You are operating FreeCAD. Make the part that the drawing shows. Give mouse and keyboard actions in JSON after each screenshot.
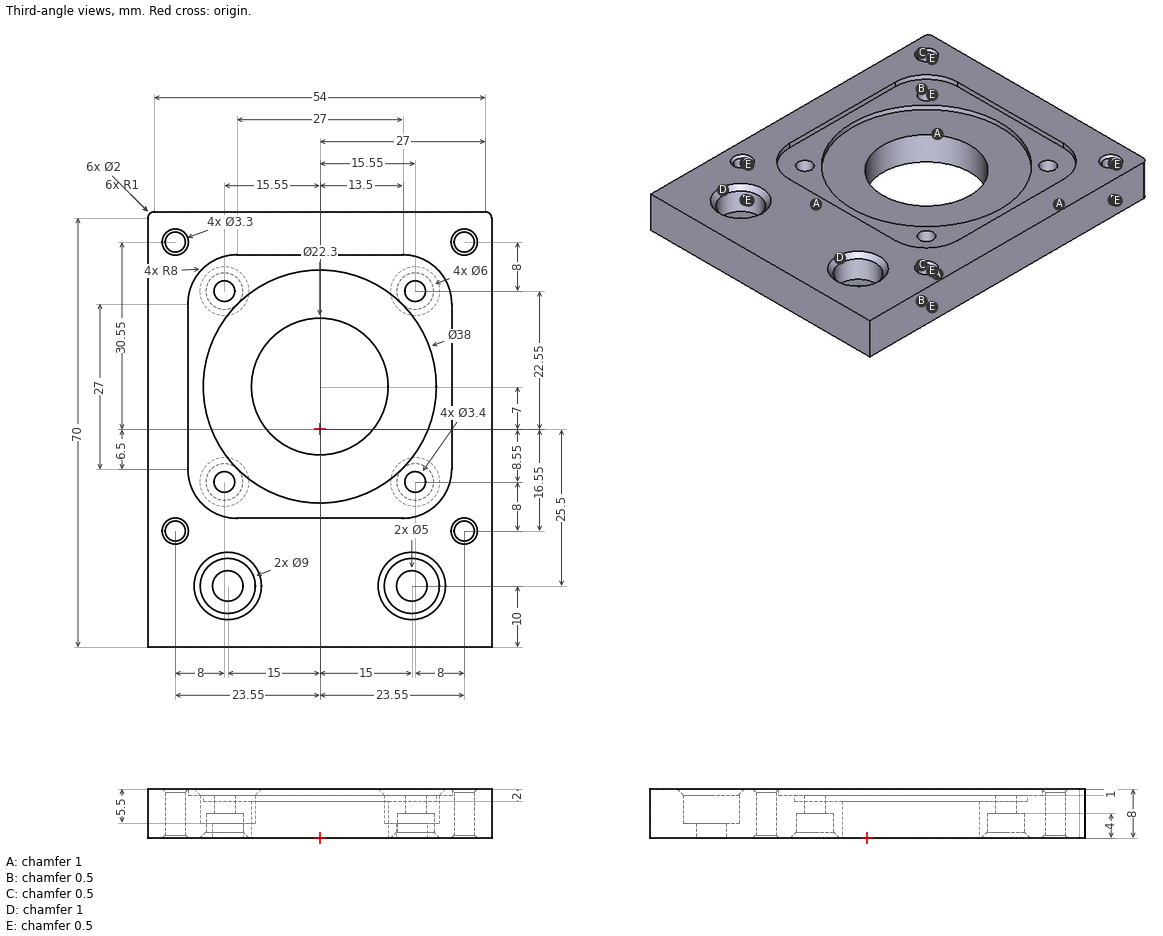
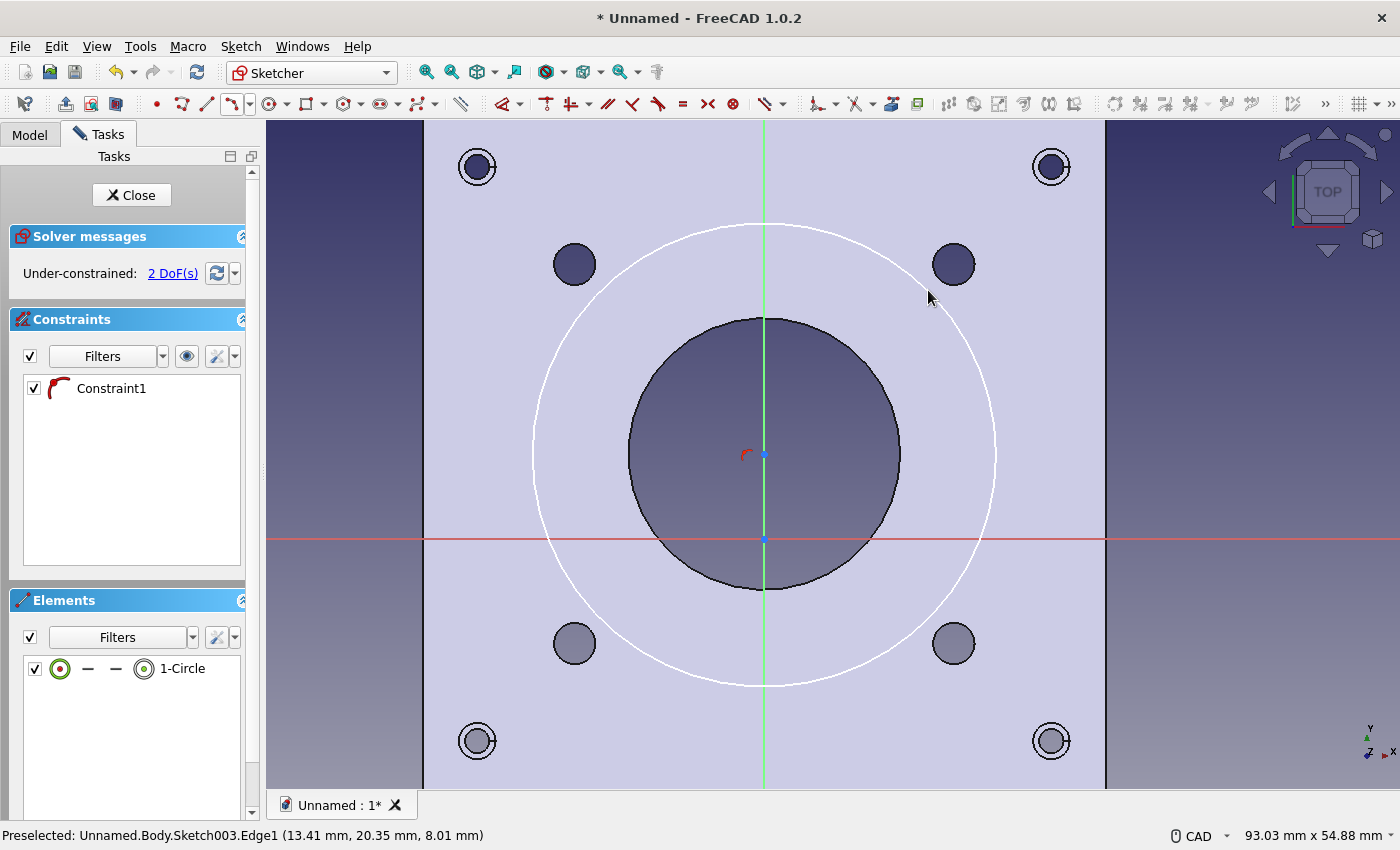
{"action": "key", "text": "d"}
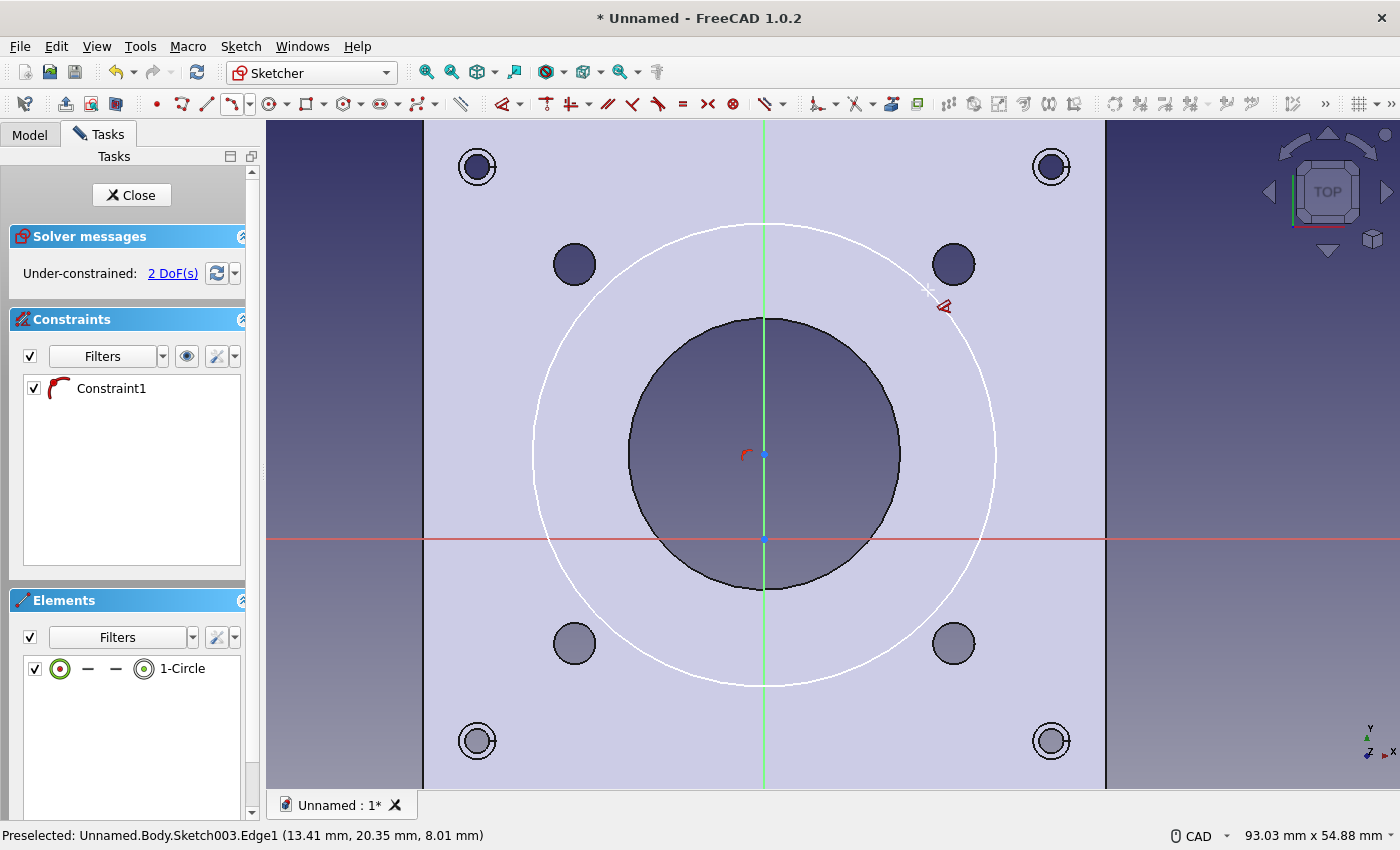
{"action": "left_click", "coordinate": [928, 291]}
{"action": "left_click", "coordinate": [951, 268]}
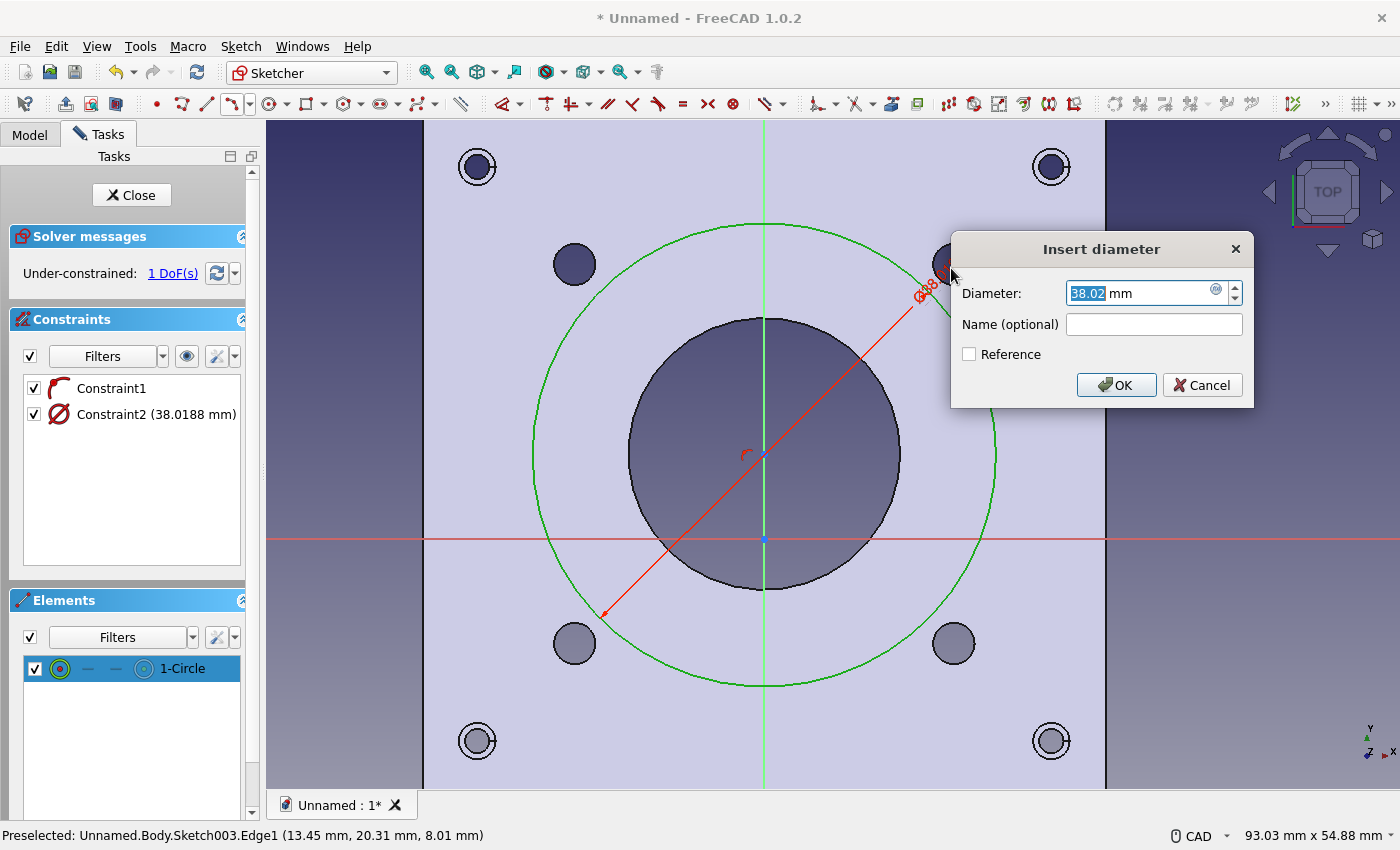
{"action": "type", "text": "38"}
{"action": "key", "text": "Return"}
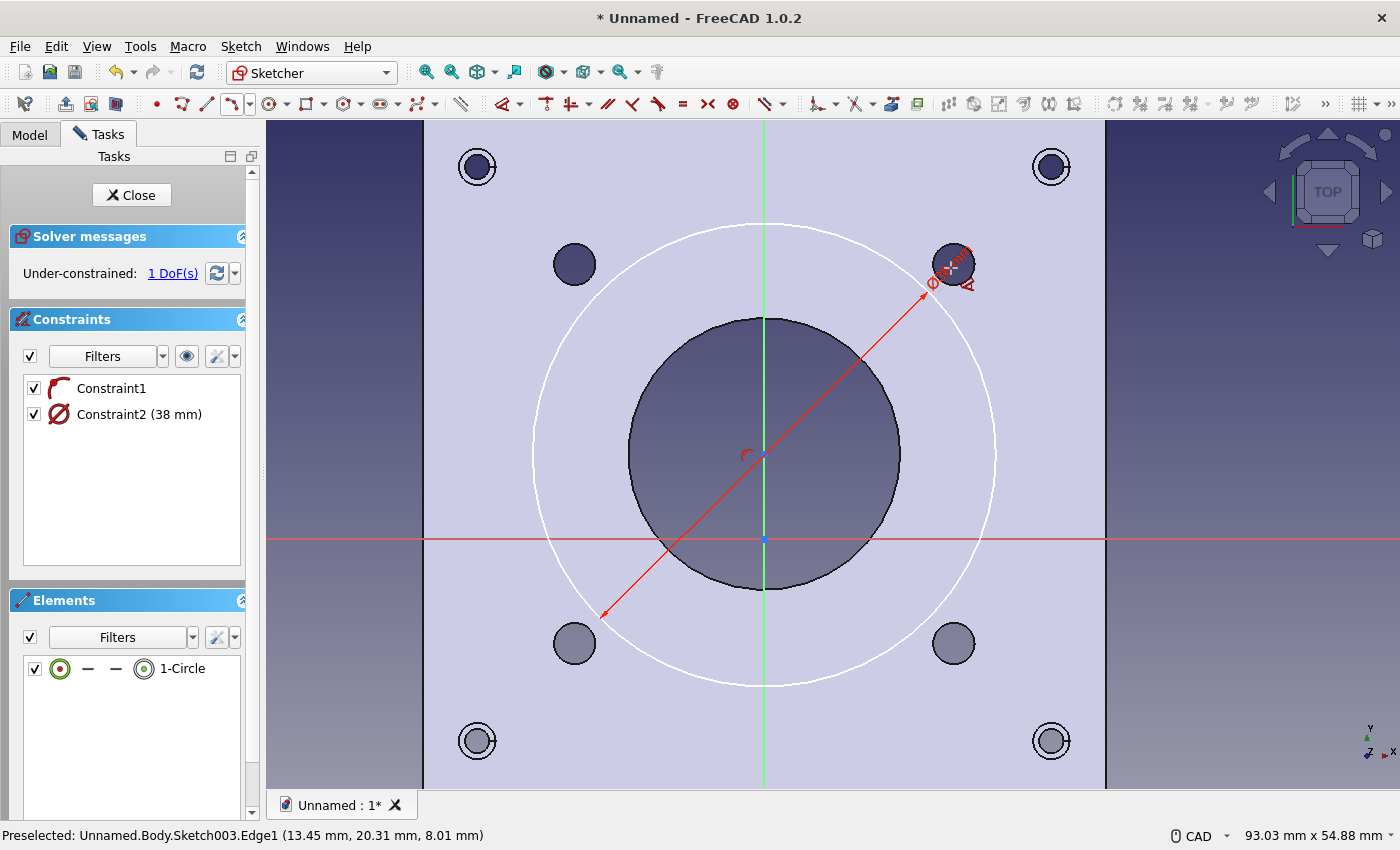
{"action": "left_click", "coordinate": [764, 455]}
{"action": "left_click", "coordinate": [798, 497]}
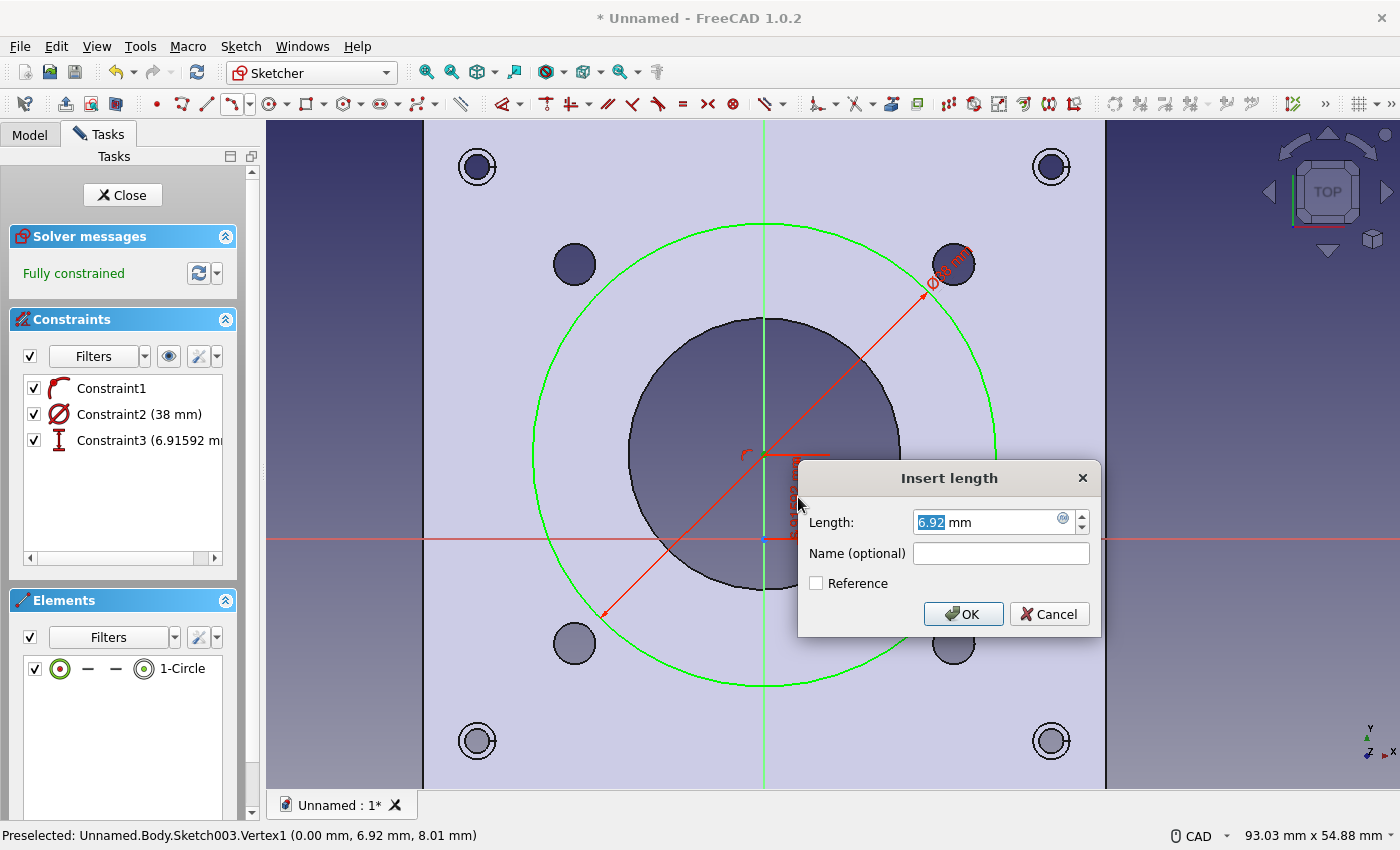
{"action": "type", "text": "7"}
{"action": "key", "text": "Return"}
{"action": "key", "text": "Escape"}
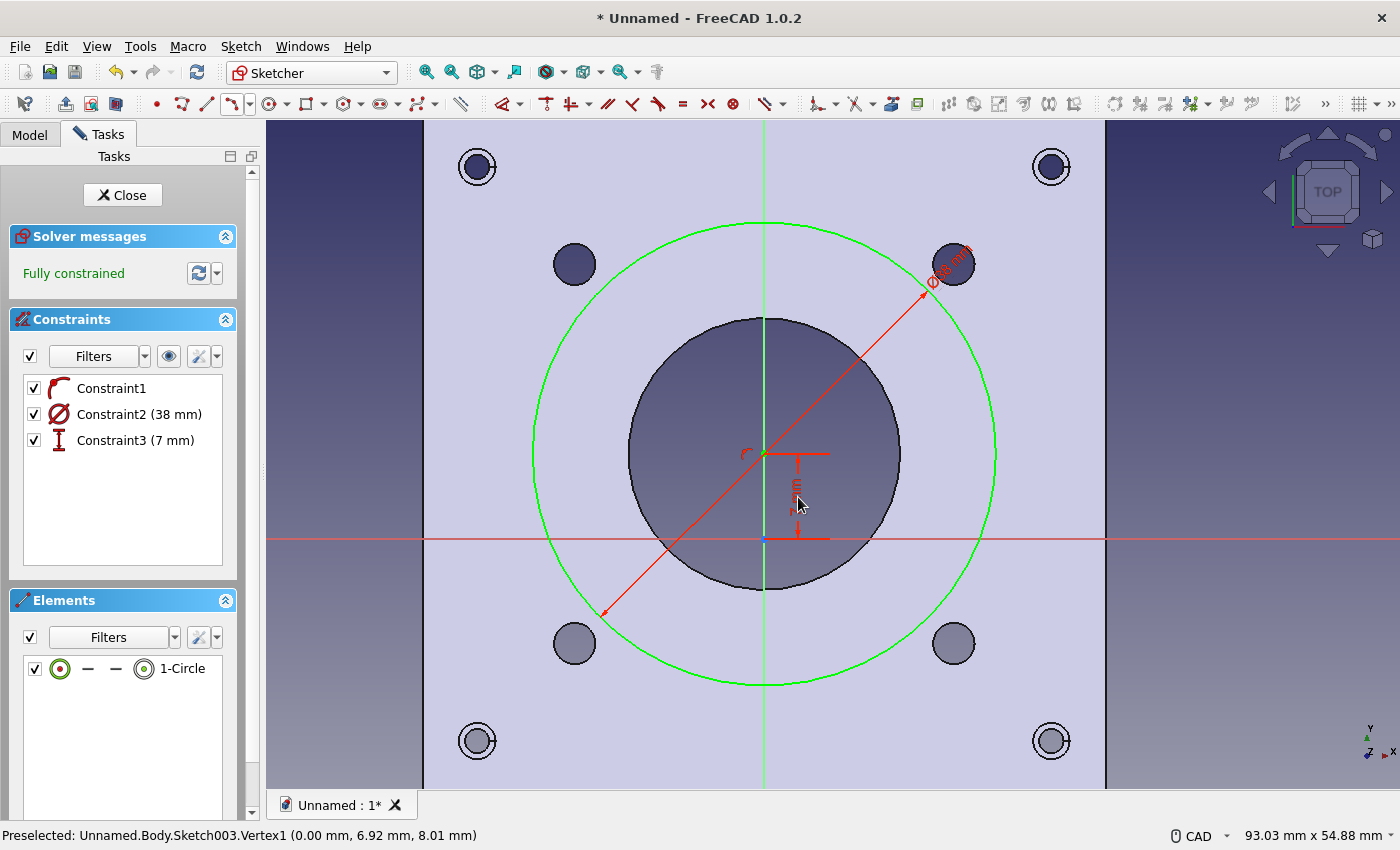
{"action": "left_click", "coordinate": [123, 195]}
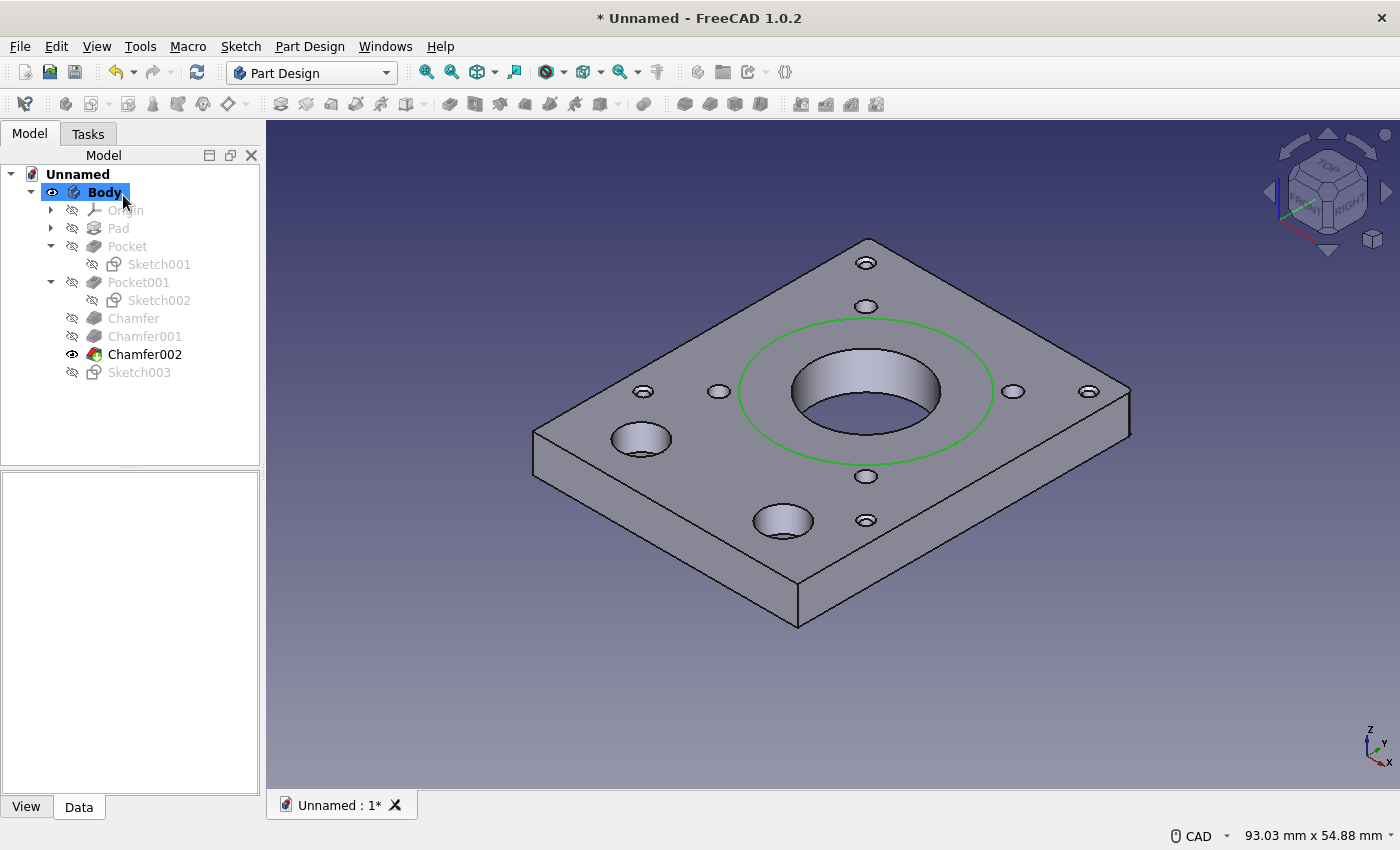
{"action": "left_click", "coordinate": [450, 104]}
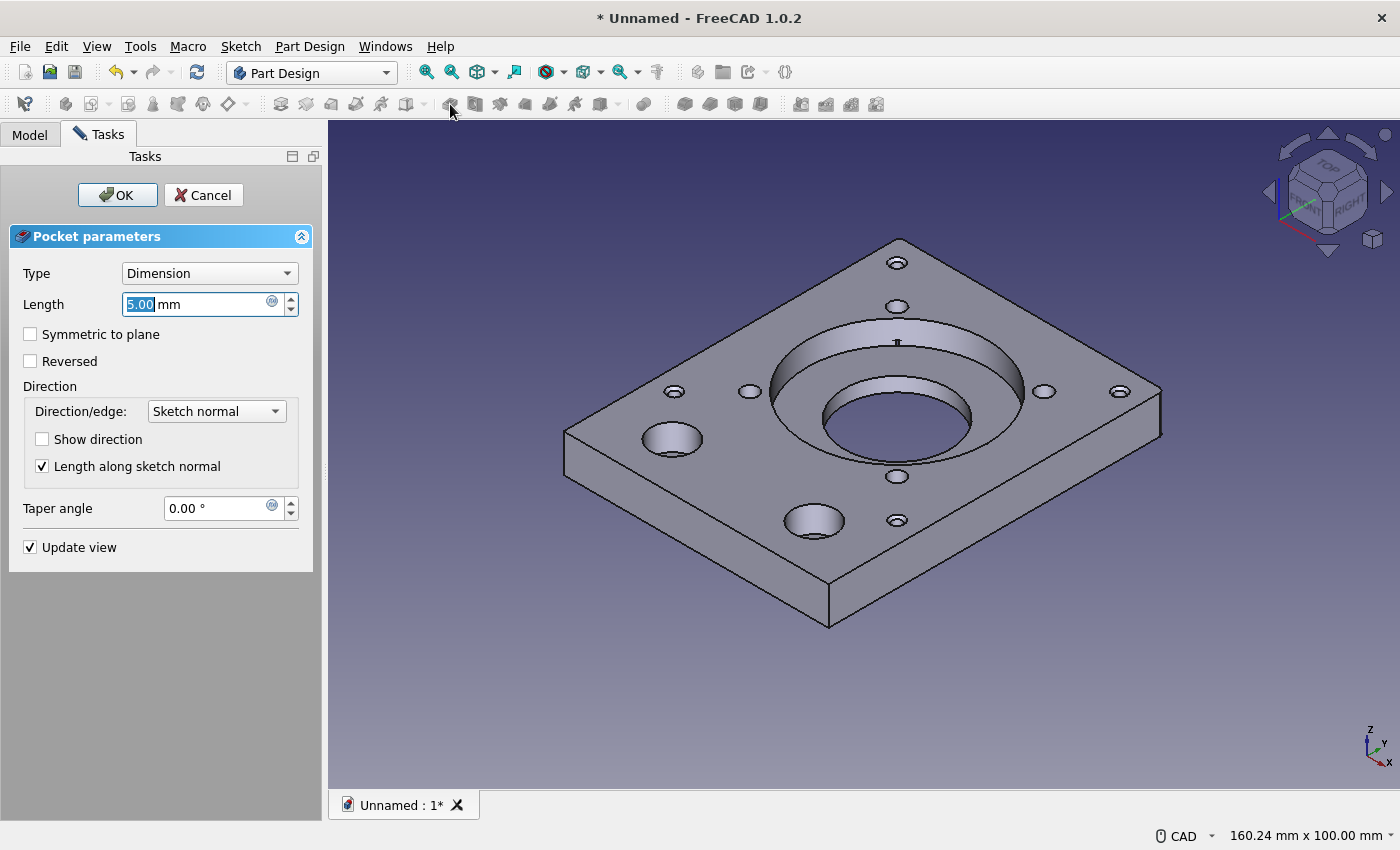
{"action": "type", "text": "2"}
{"action": "key", "text": "Tab"}